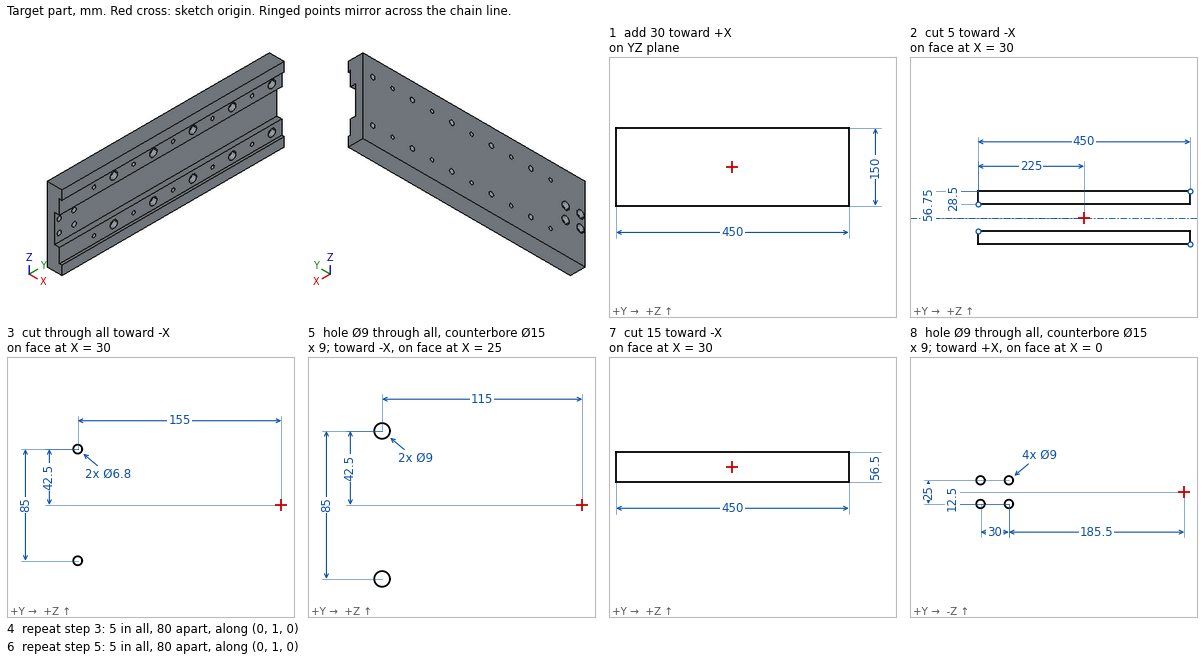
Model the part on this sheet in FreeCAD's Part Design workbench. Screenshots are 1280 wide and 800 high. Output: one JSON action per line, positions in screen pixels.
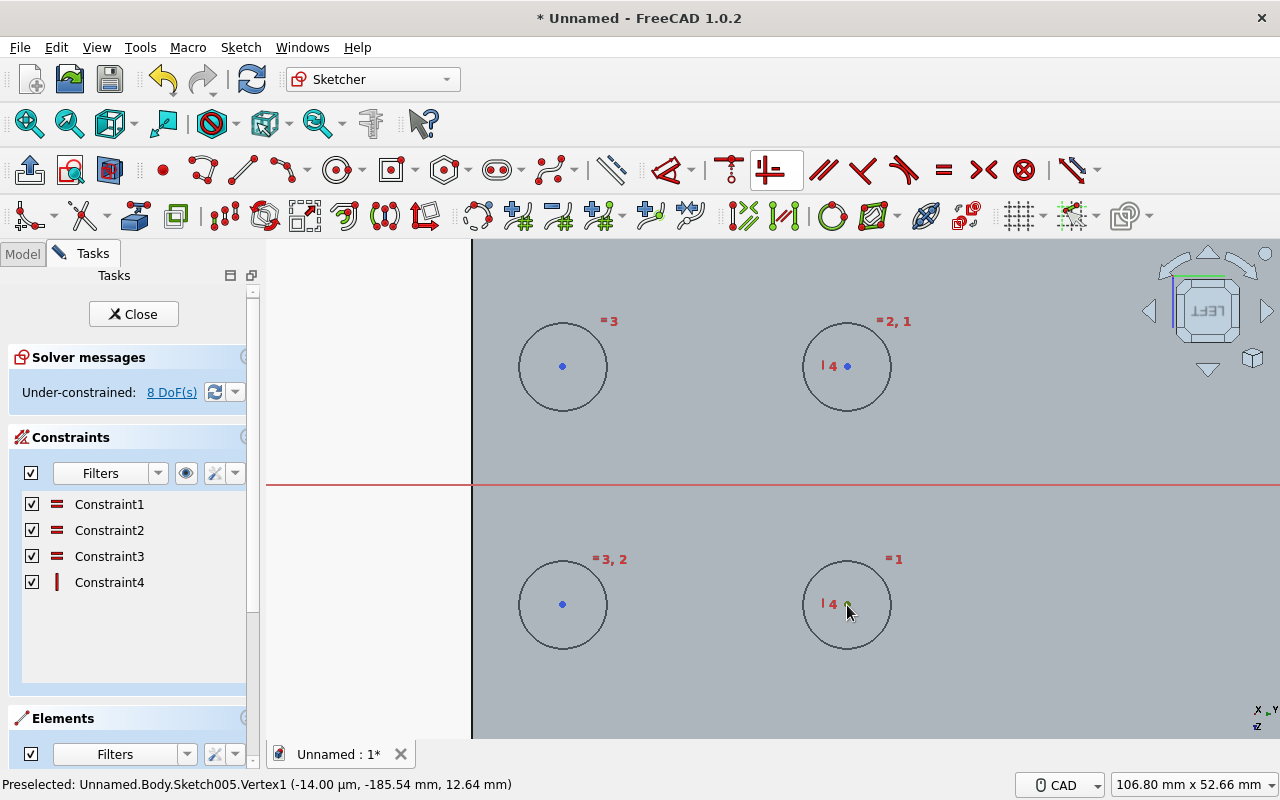
{"action": "left_click", "coordinate": [563, 605]}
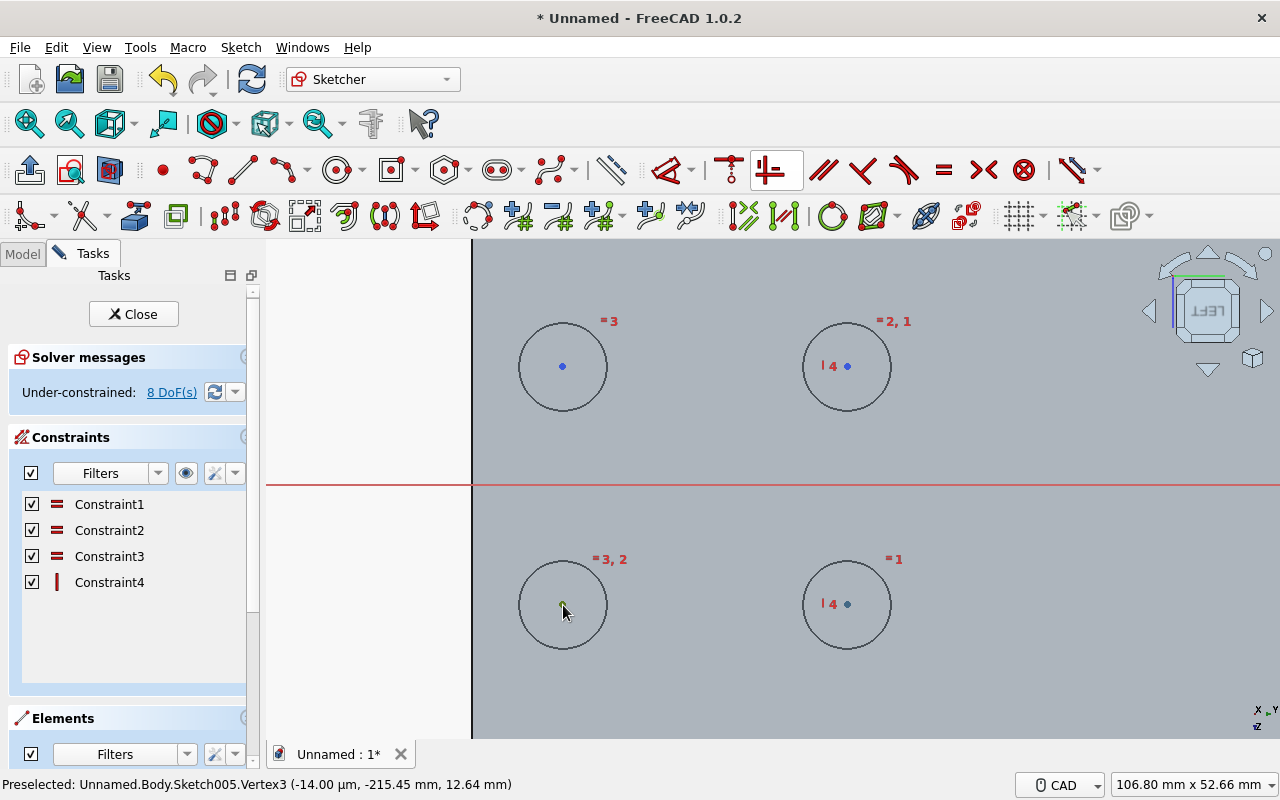
{"action": "key", "text": "h"}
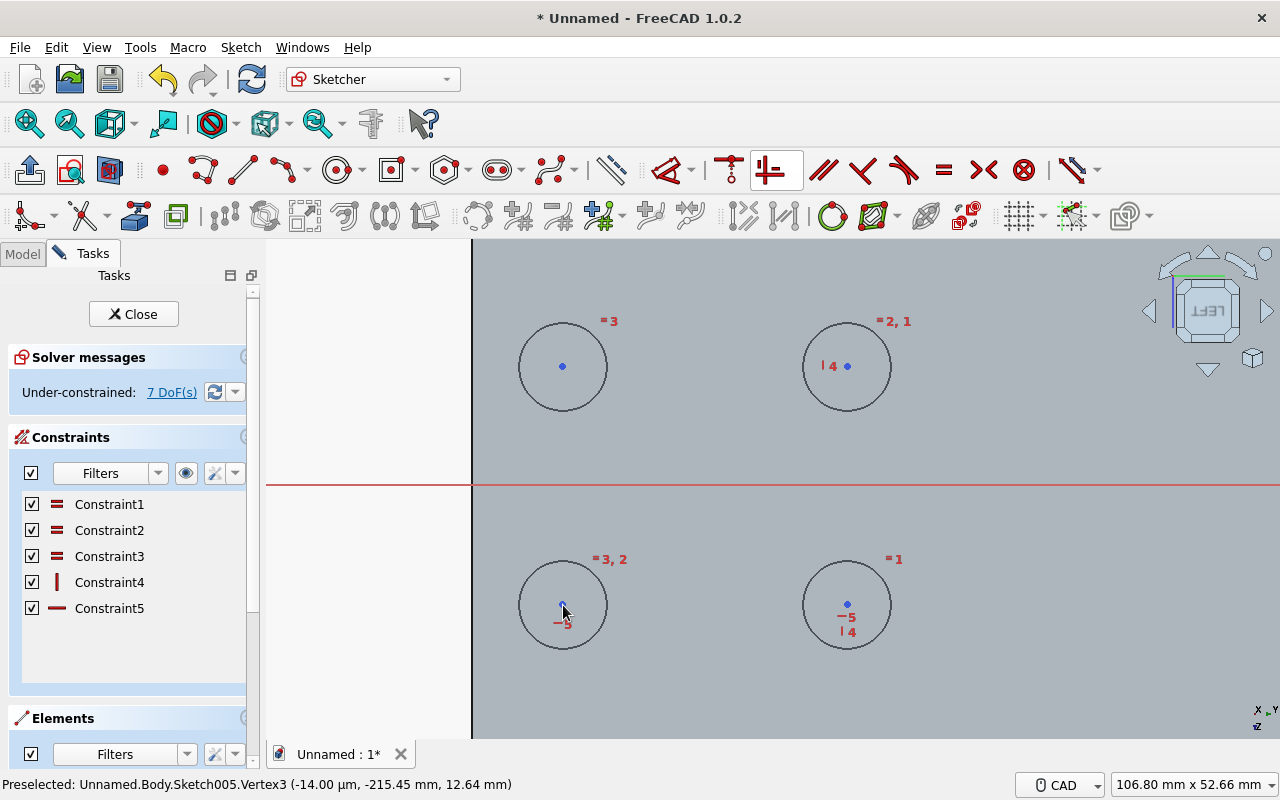
{"action": "left_click", "coordinate": [563, 605]}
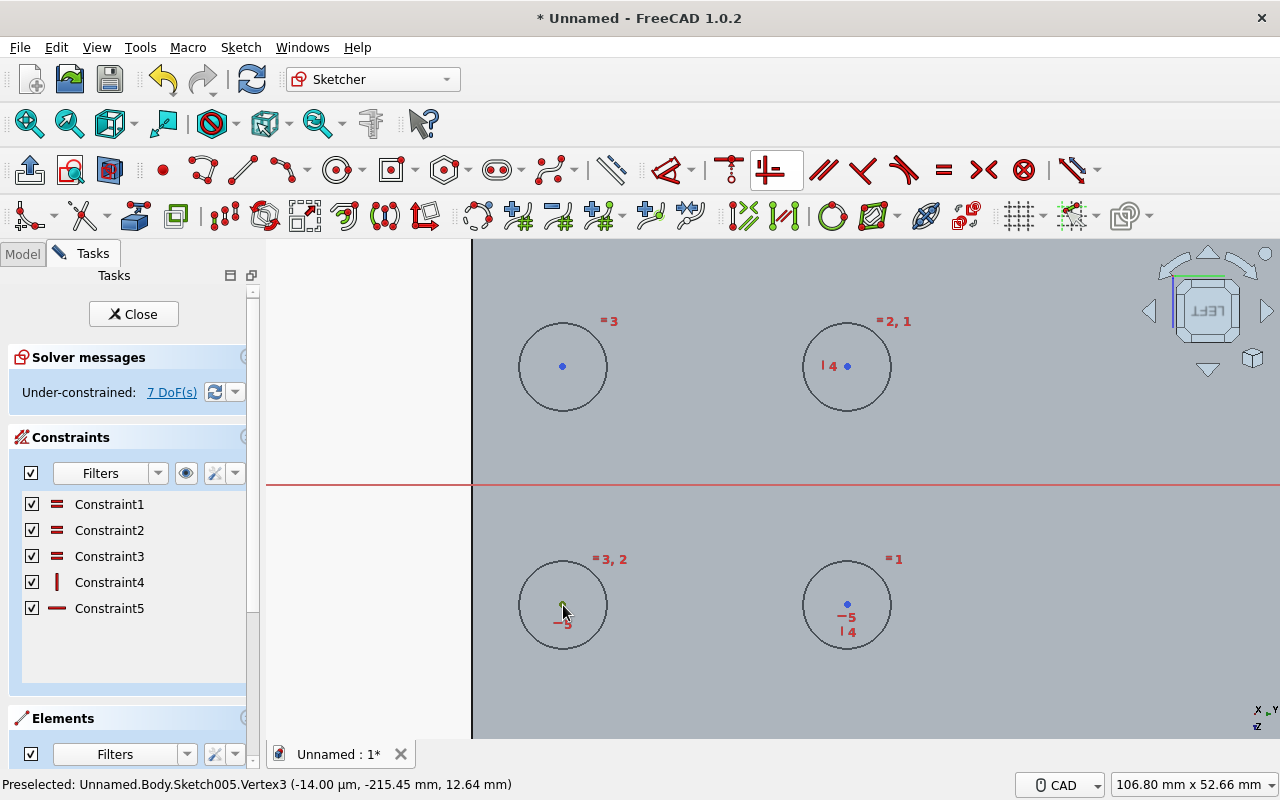
{"action": "left_click", "coordinate": [563, 367]}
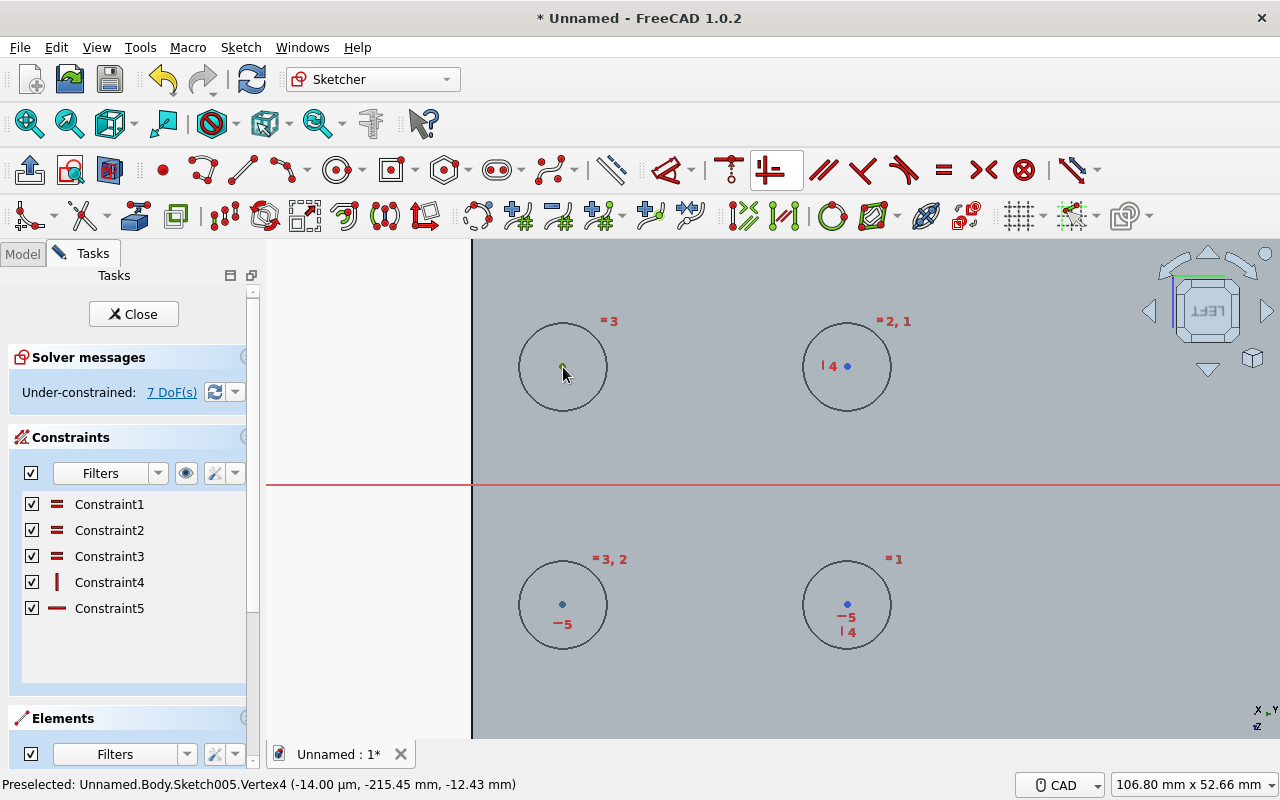
{"action": "key", "text": "v"}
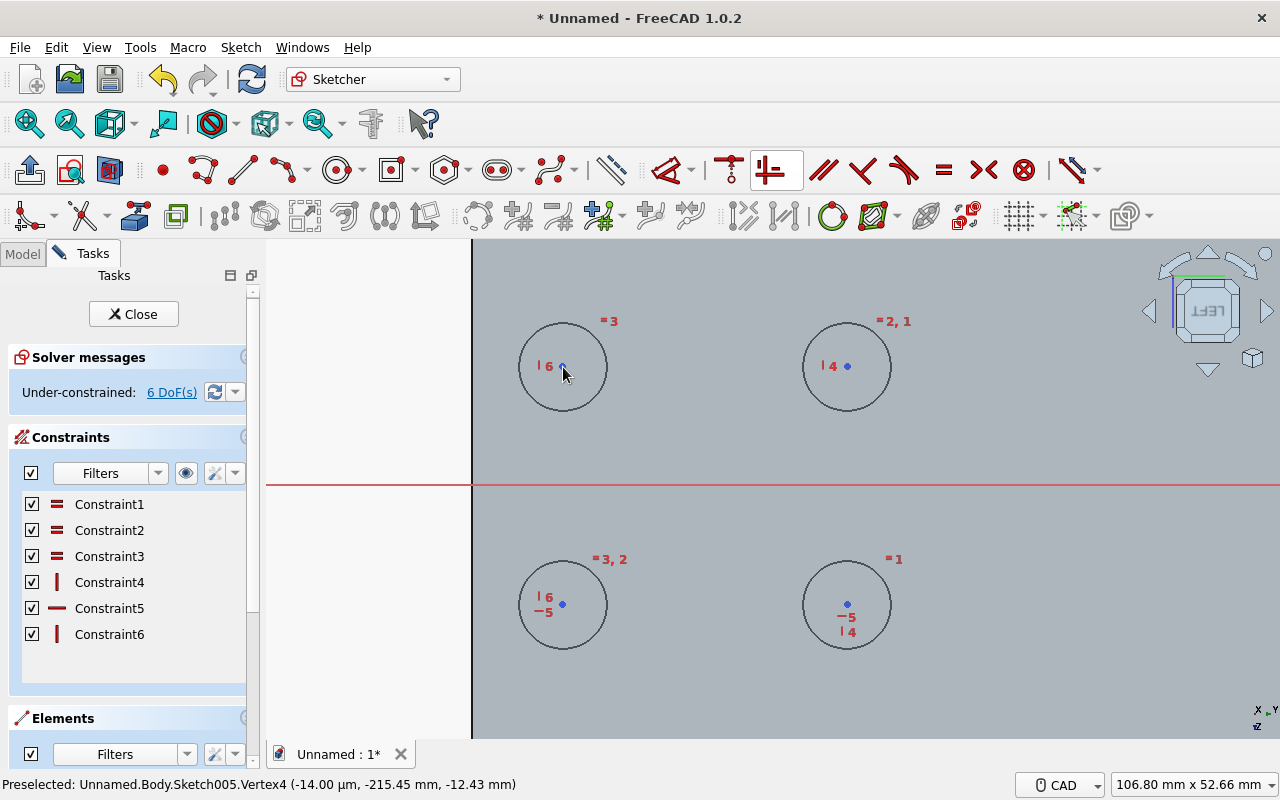
{"action": "left_click", "coordinate": [847, 367]}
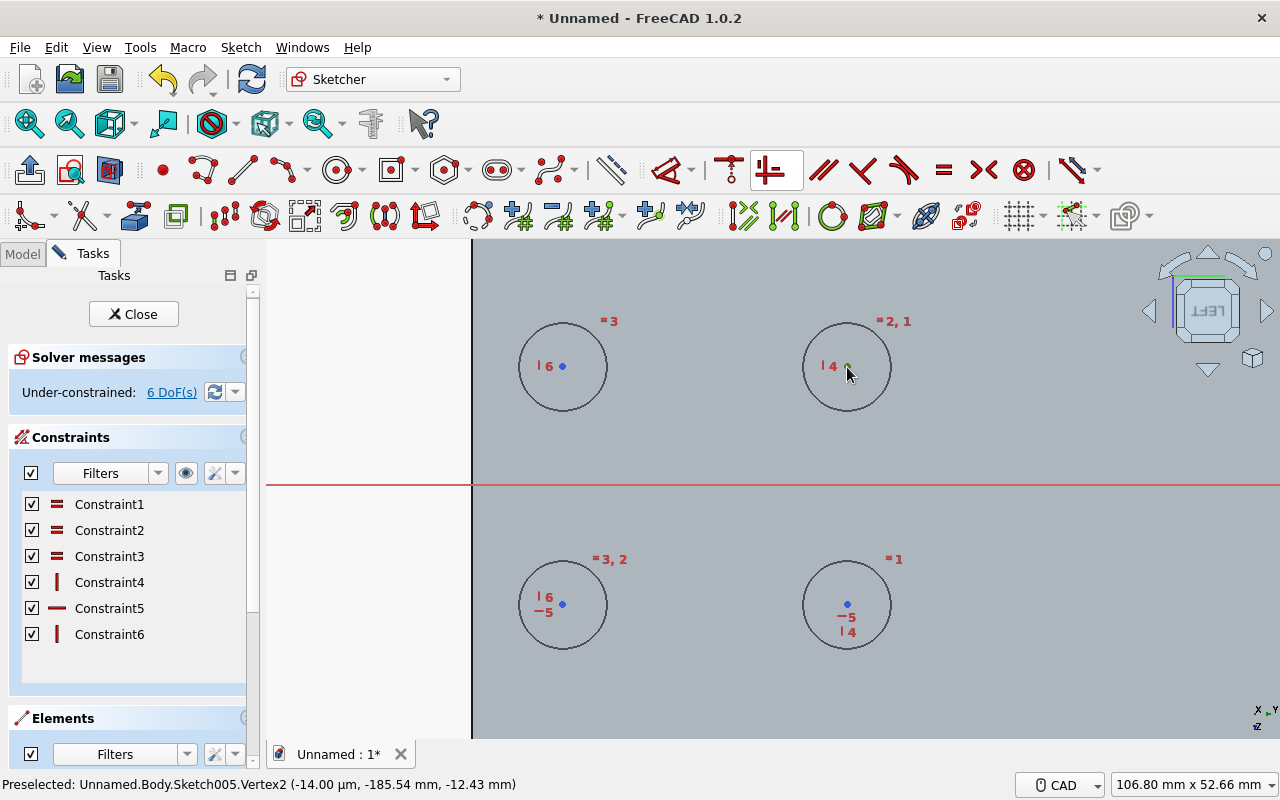
{"action": "left_click", "coordinate": [563, 367]}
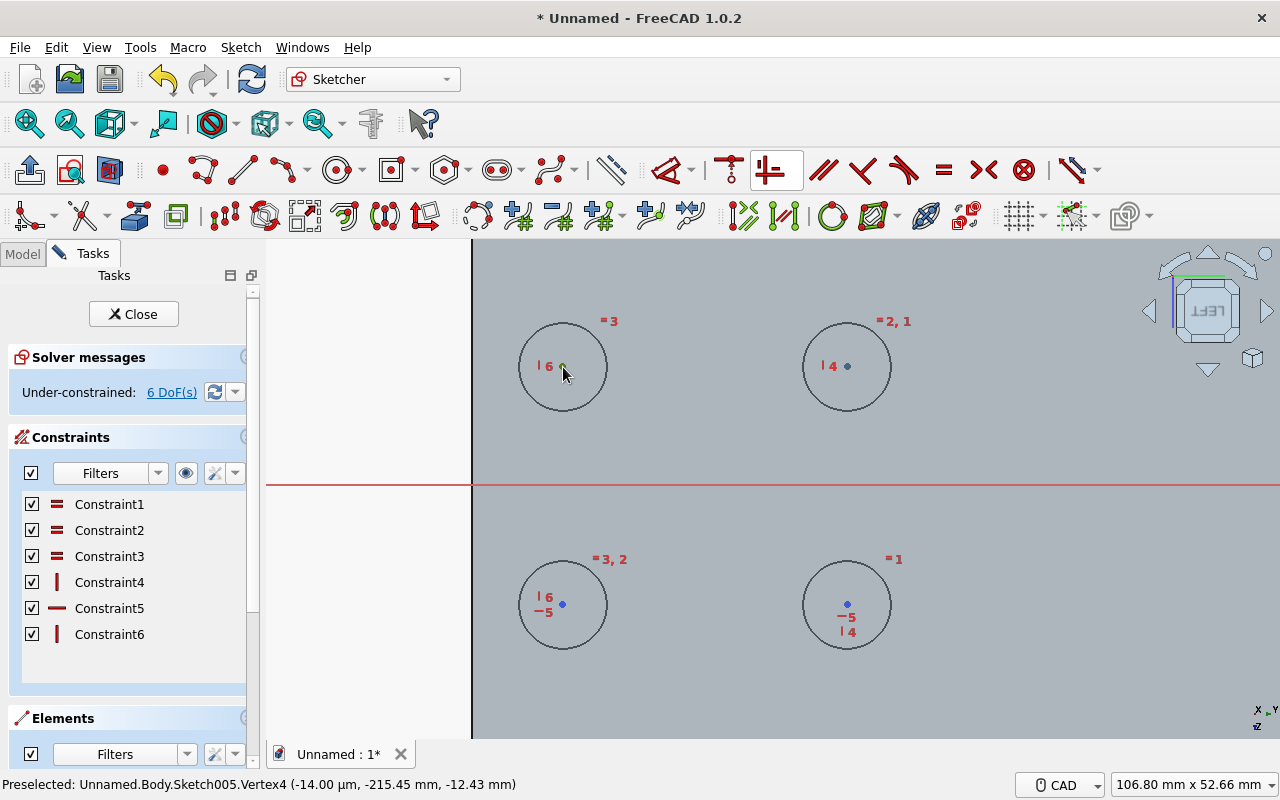
{"action": "left_click", "coordinate": [798, 170]}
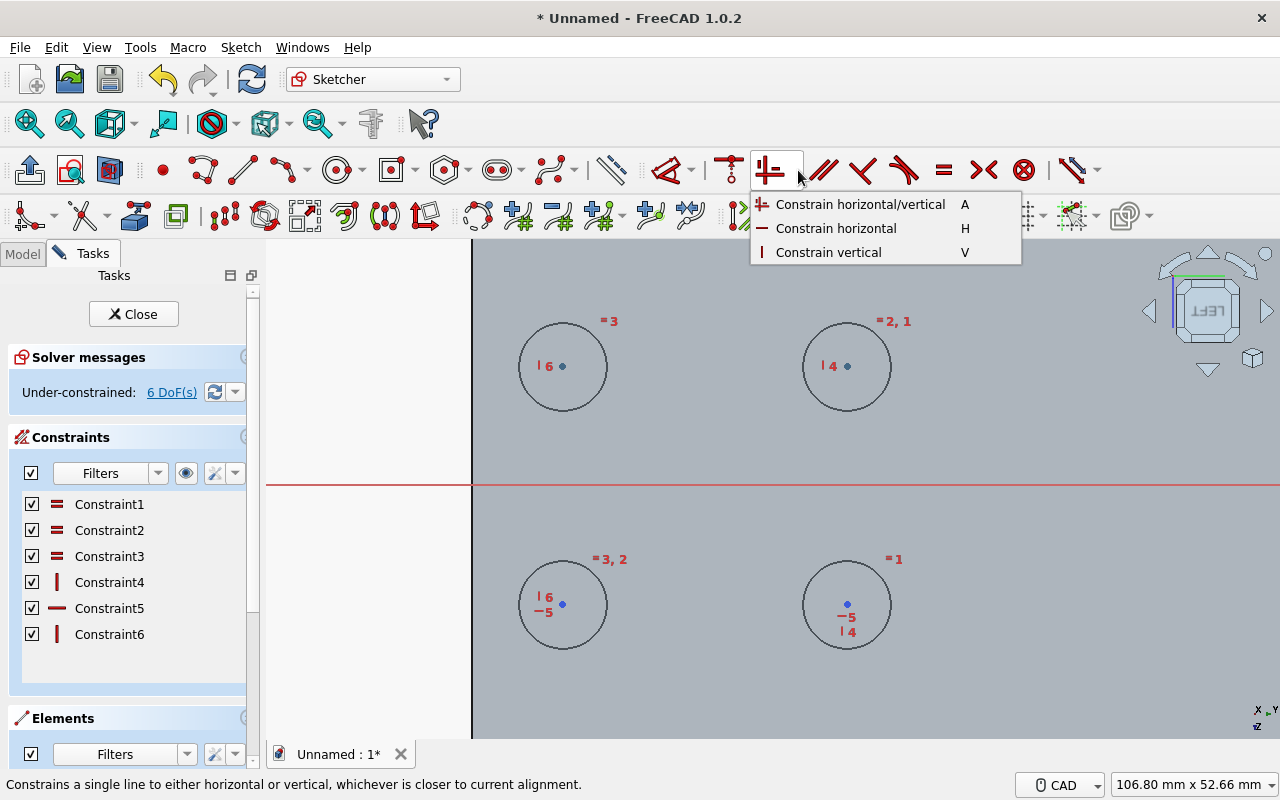
{"action": "left_click", "coordinate": [886, 228]}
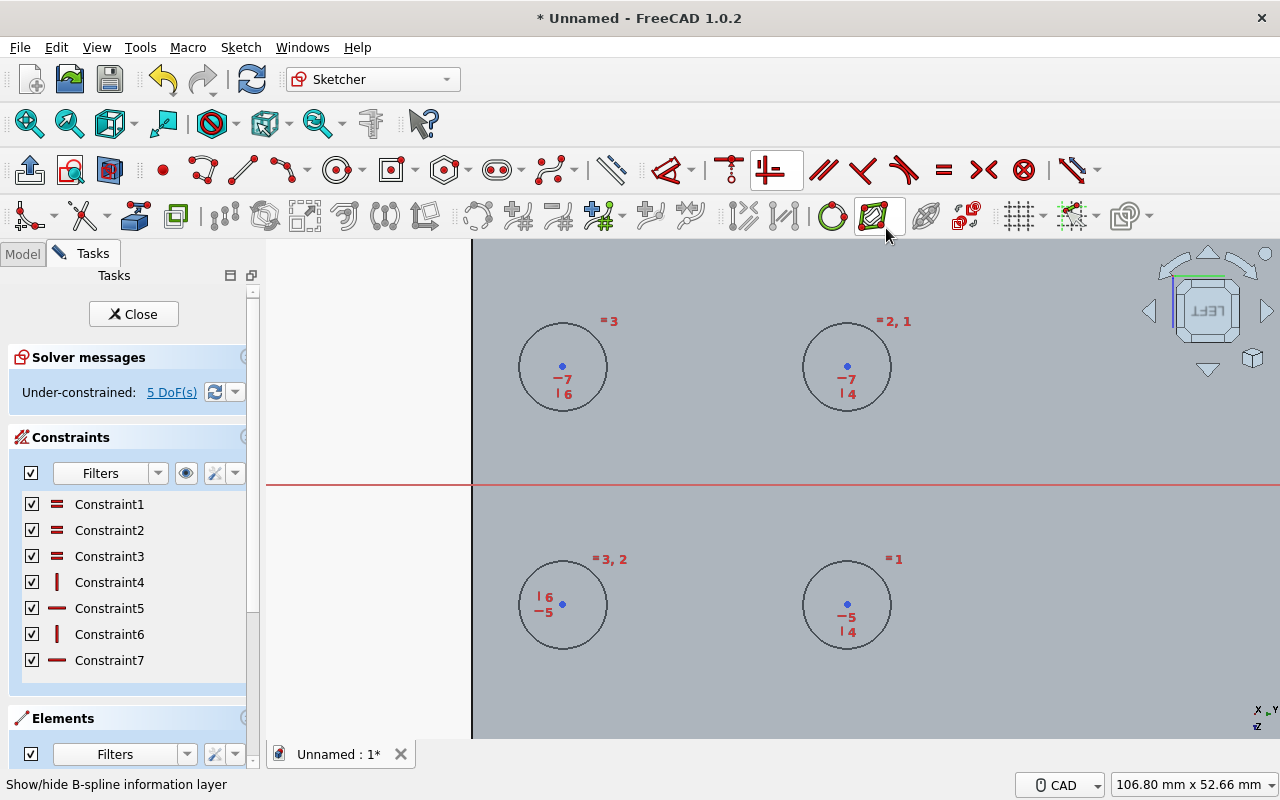
{"action": "left_click", "coordinate": [666, 170]}